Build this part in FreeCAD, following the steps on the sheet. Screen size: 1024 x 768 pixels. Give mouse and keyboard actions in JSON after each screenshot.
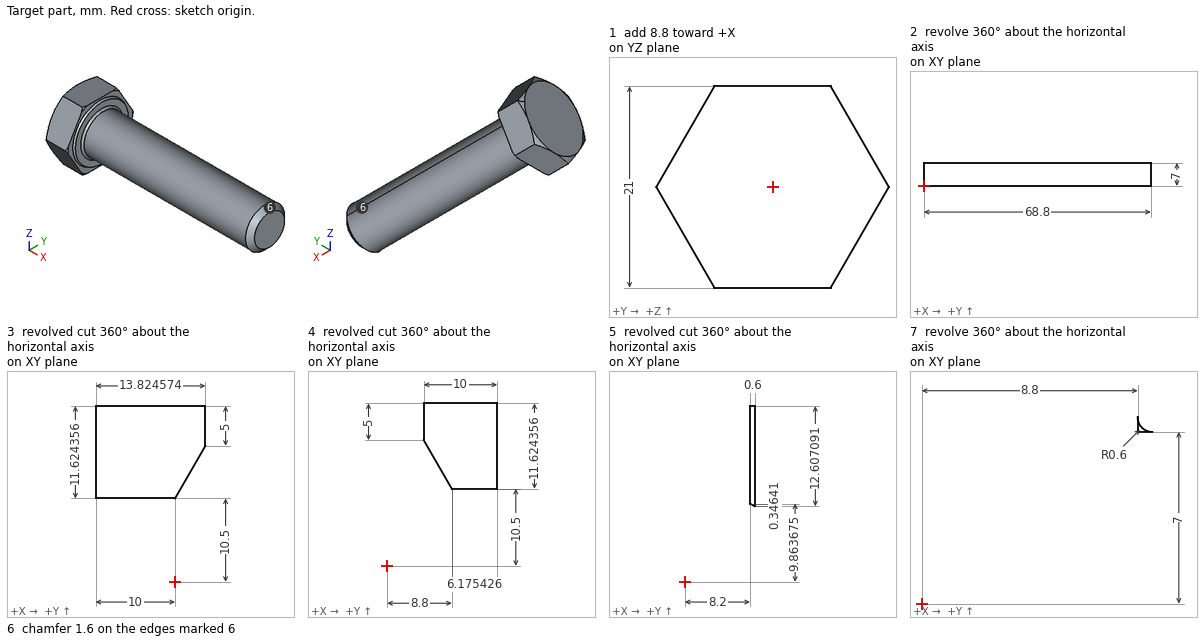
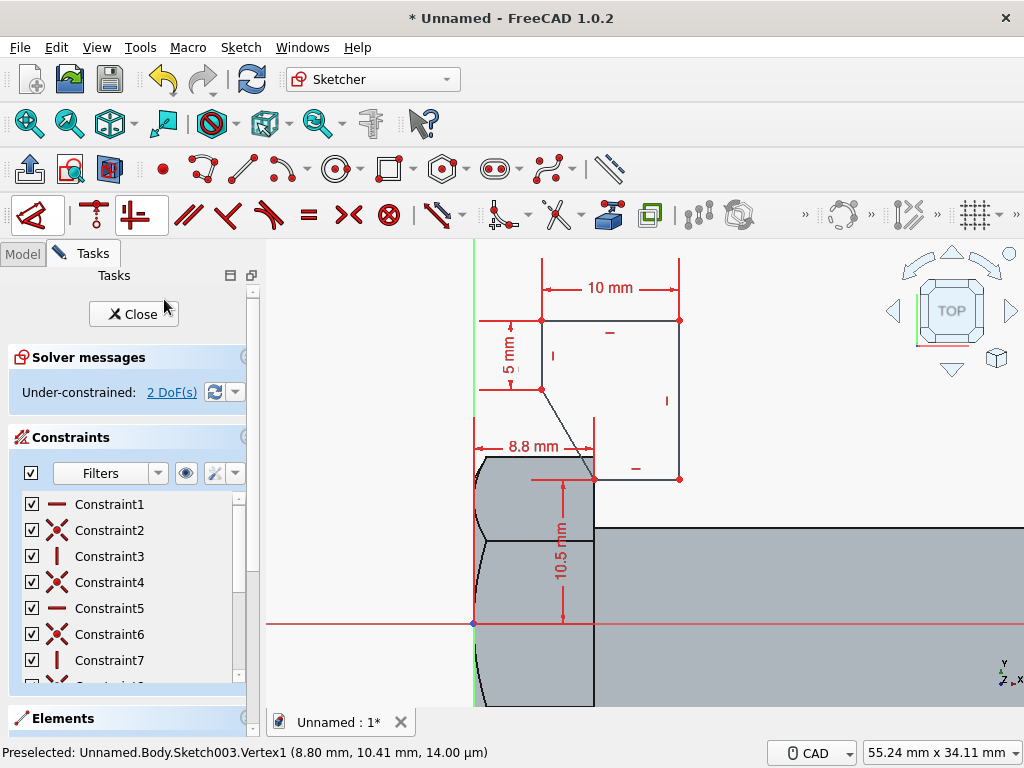
{"action": "left_click", "coordinate": [620, 480]}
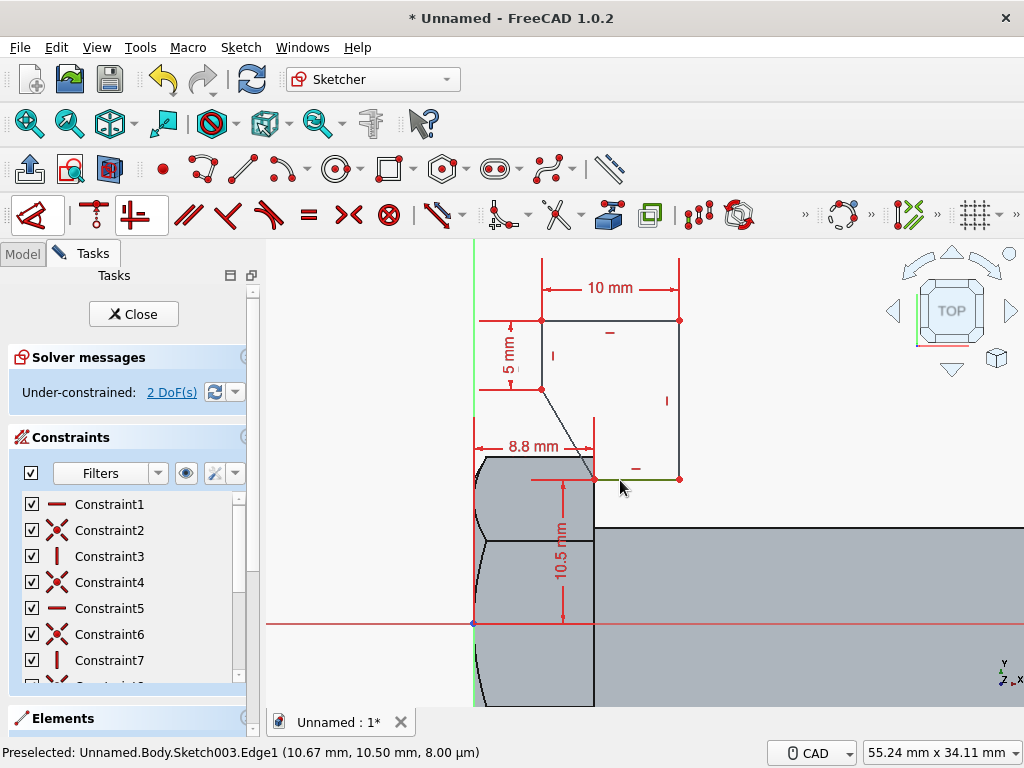
{"action": "left_click", "coordinate": [58, 216]}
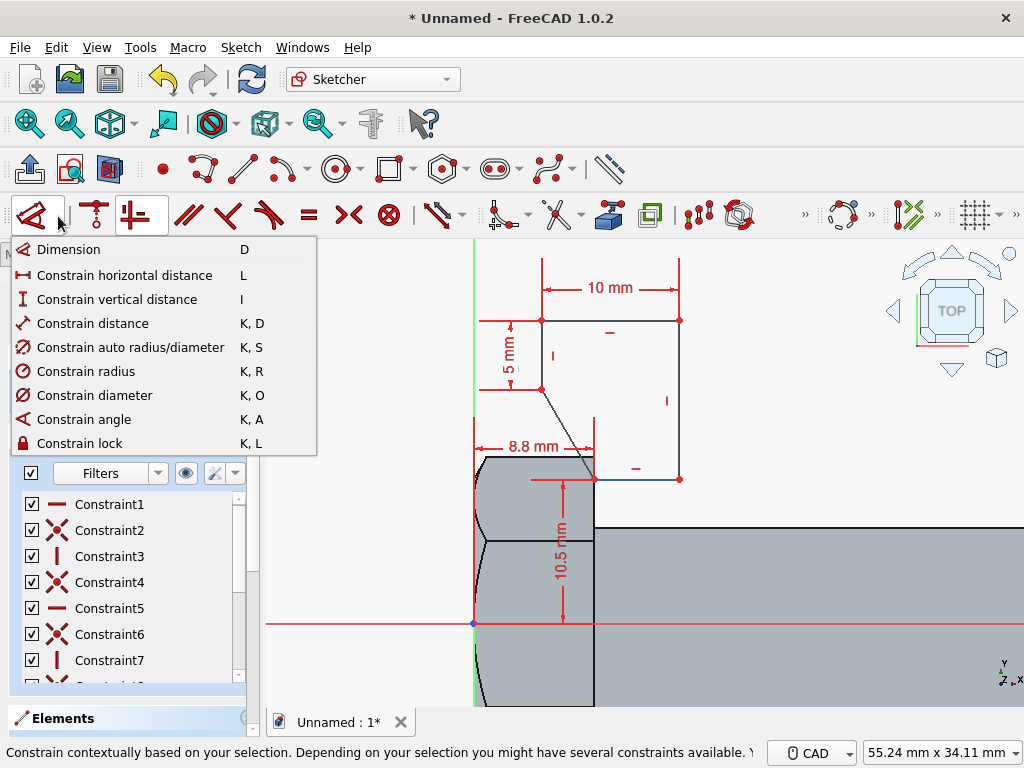
{"action": "left_click", "coordinate": [164, 275]}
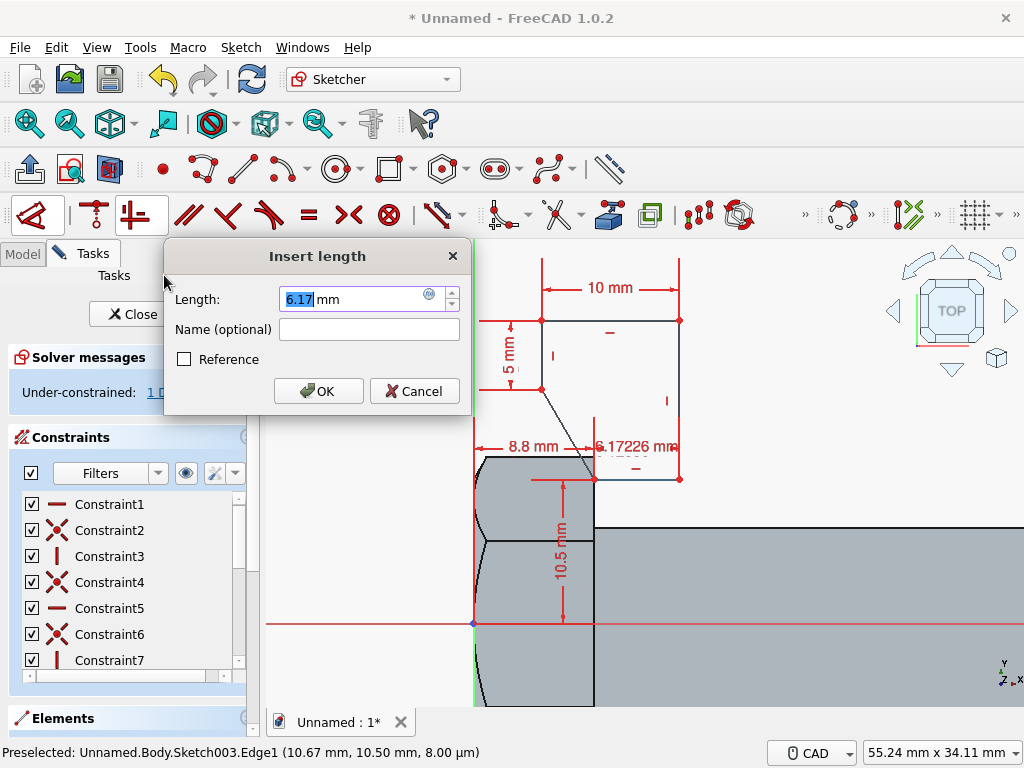
{"action": "type", "text": "6.175426"}
{"action": "key", "text": "Return"}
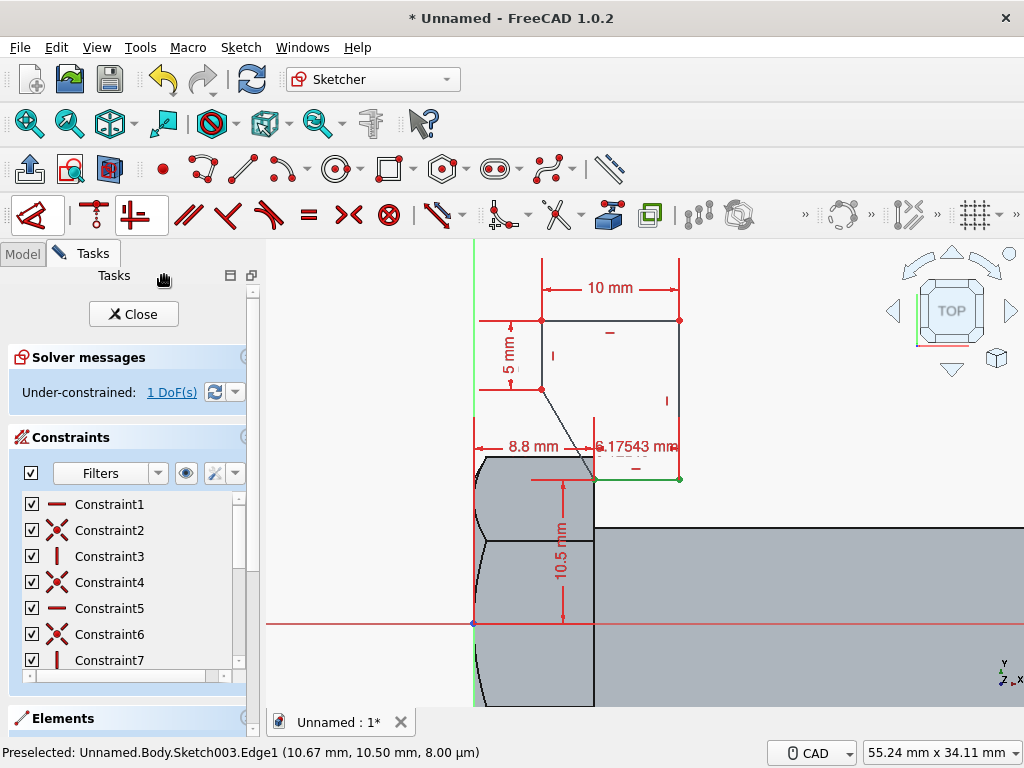
{"action": "left_click", "coordinate": [679, 432]}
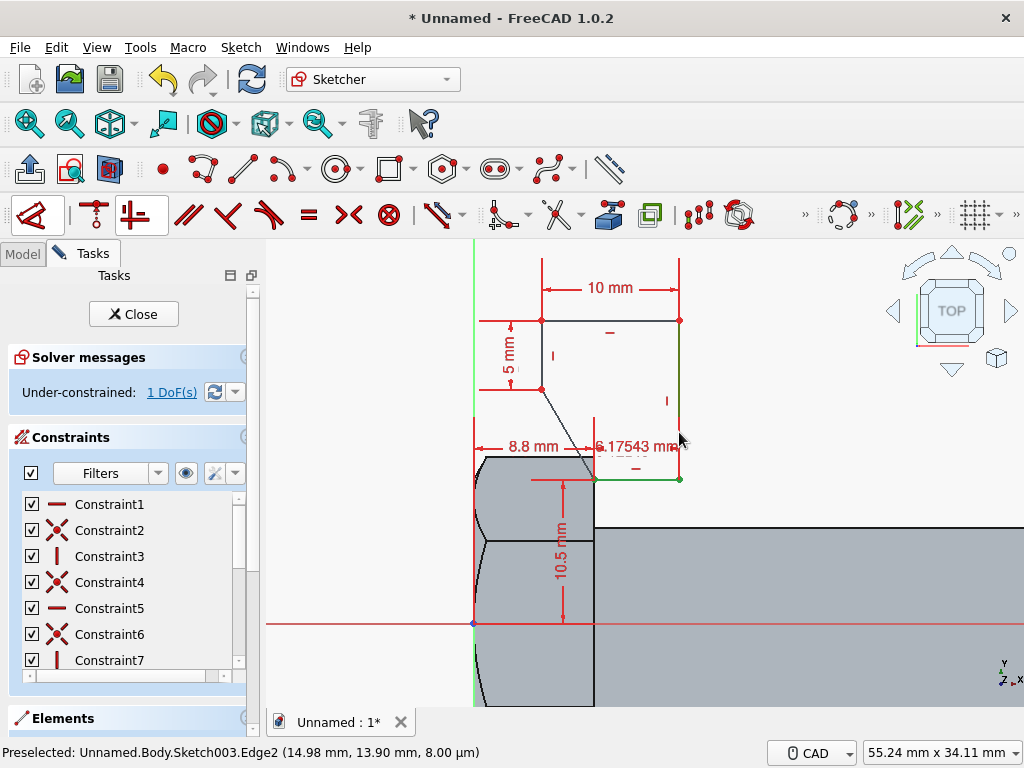
{"action": "key", "text": "i"}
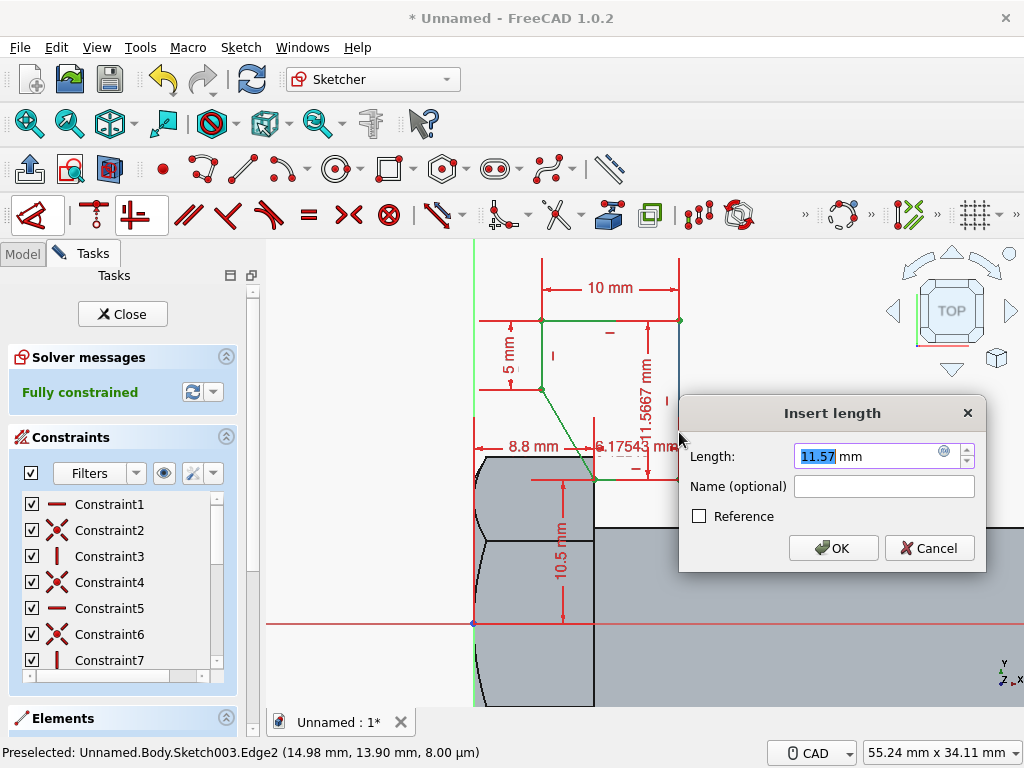
{"action": "type", "text": "11.624356"}
{"action": "key", "text": "Return"}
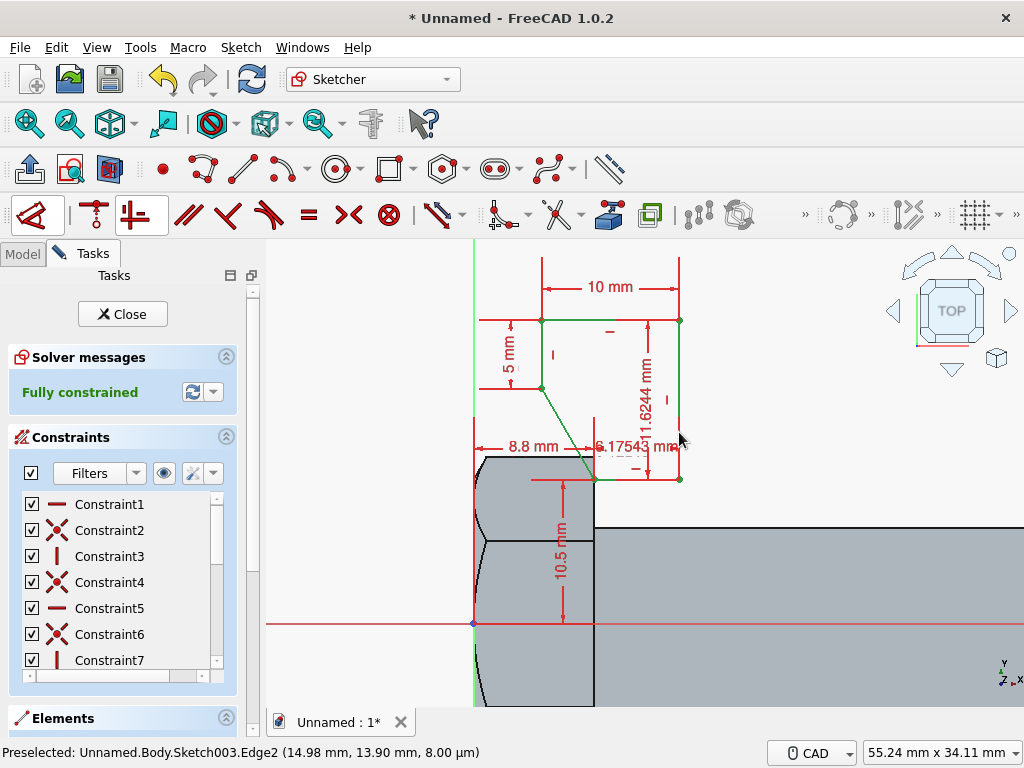
{"action": "left_click", "coordinate": [123, 314]}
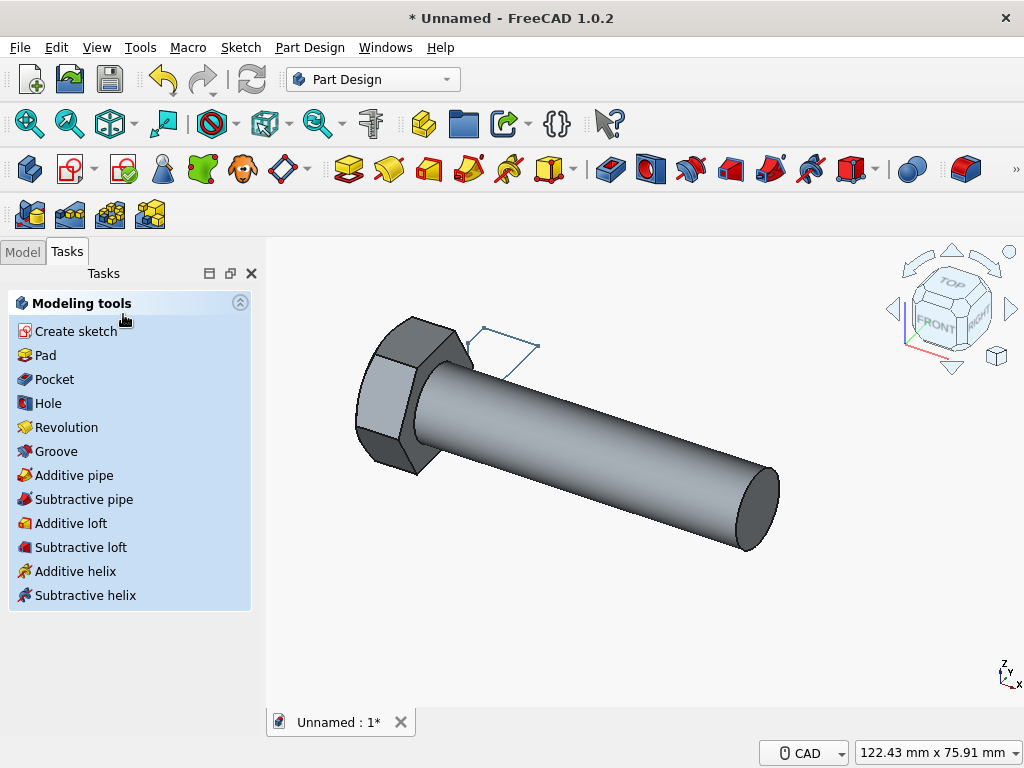
{"action": "left_click", "coordinate": [692, 170]}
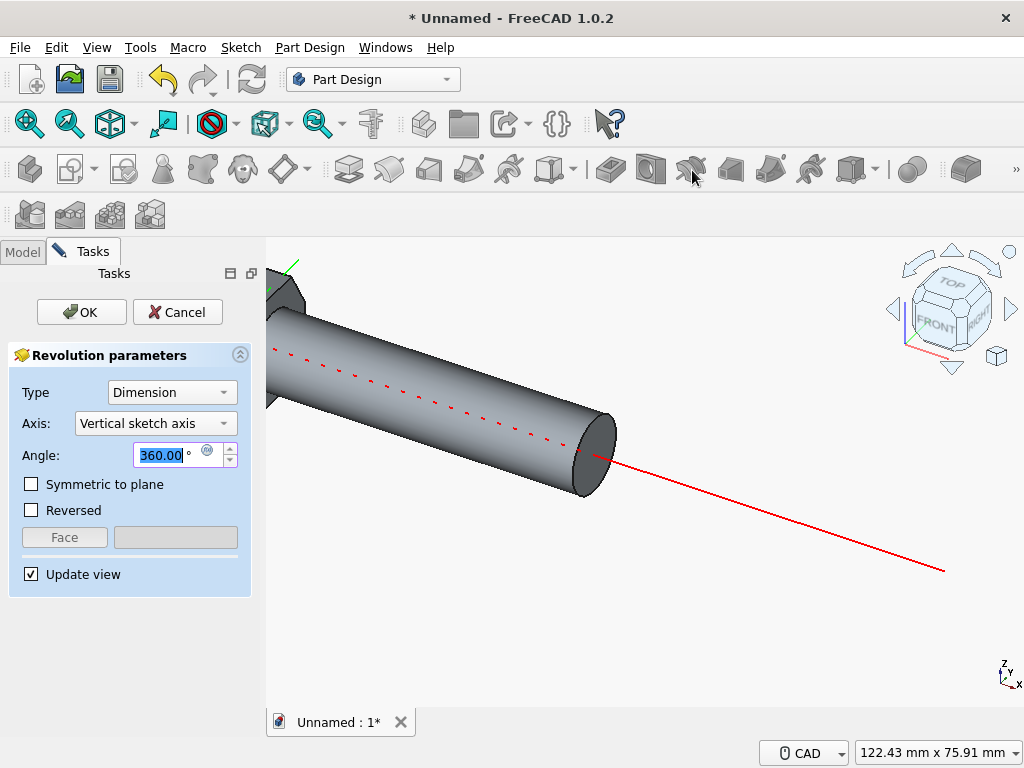
{"action": "left_click", "coordinate": [156, 424]}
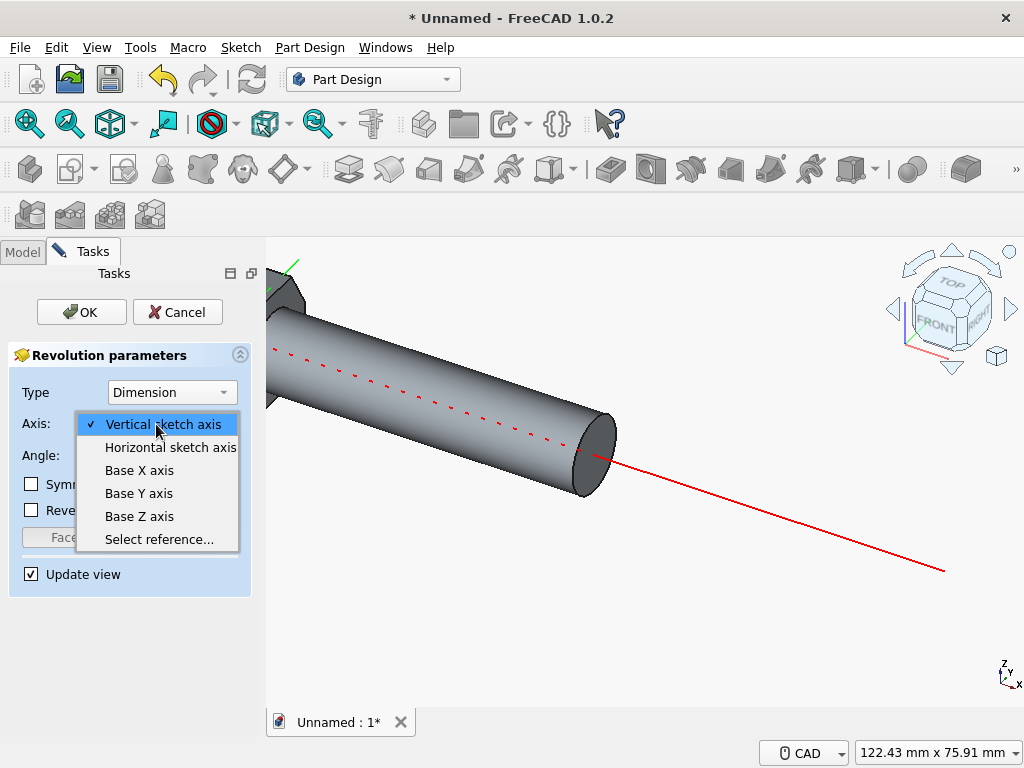
{"action": "left_click", "coordinate": [156, 448]}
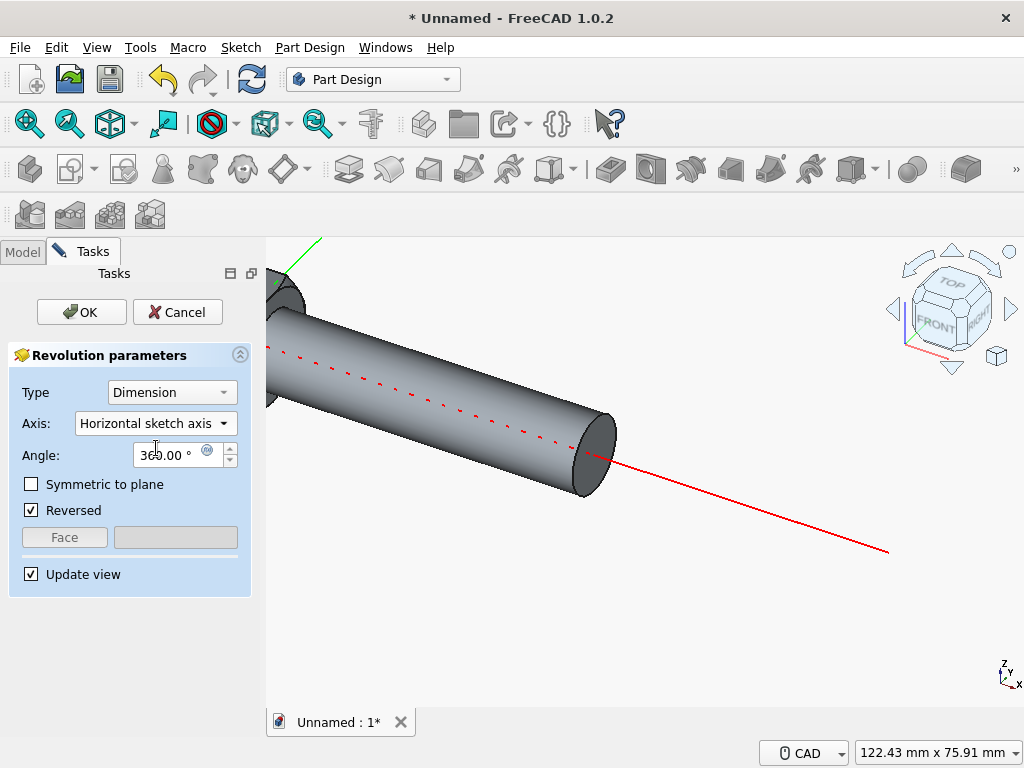
{"action": "left_click", "coordinate": [82, 312]}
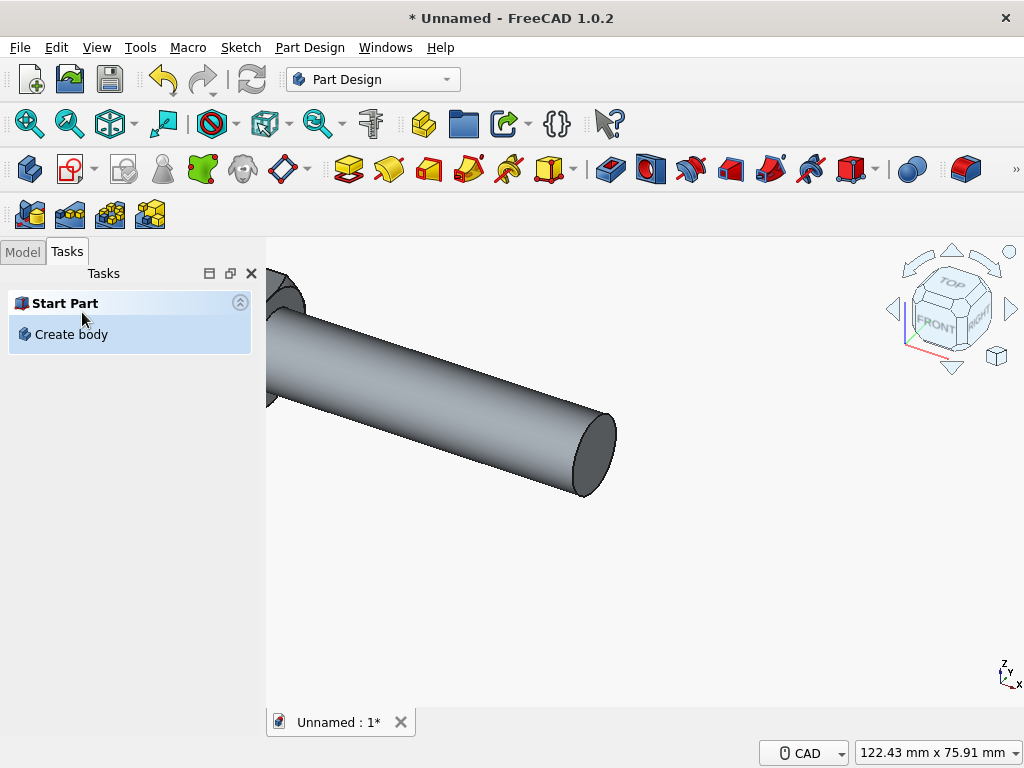
{"action": "key", "text": "v f"}